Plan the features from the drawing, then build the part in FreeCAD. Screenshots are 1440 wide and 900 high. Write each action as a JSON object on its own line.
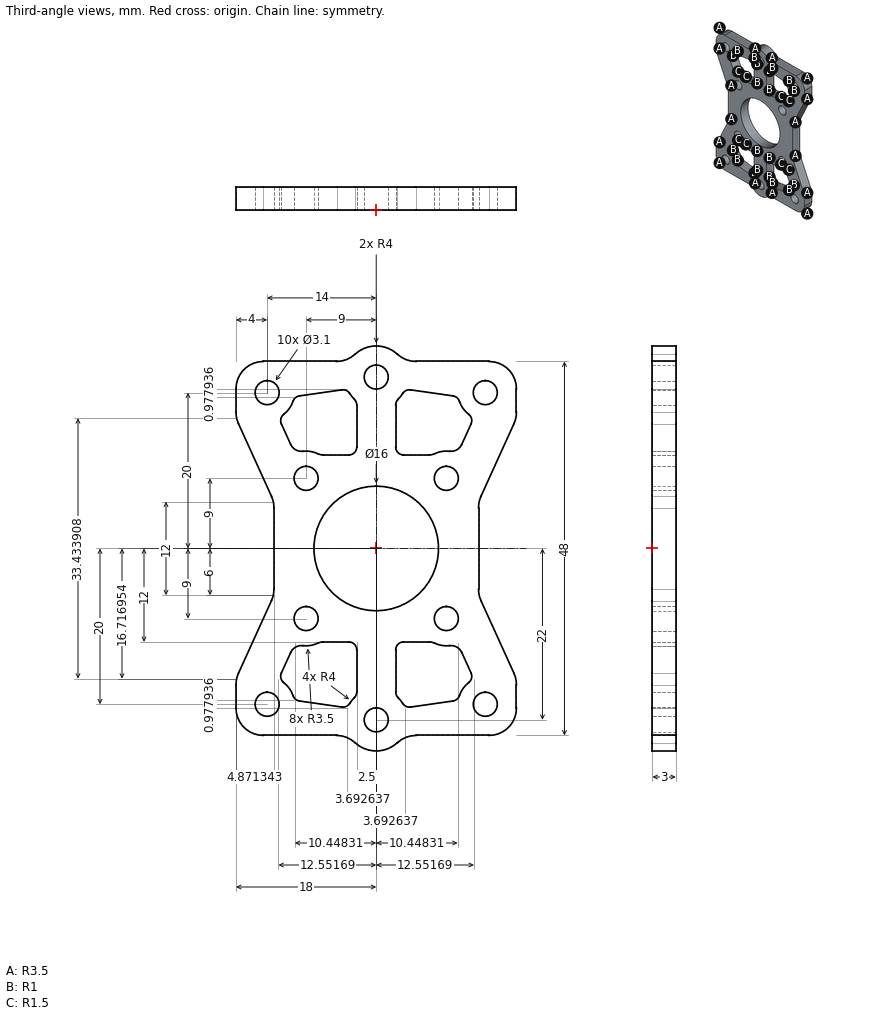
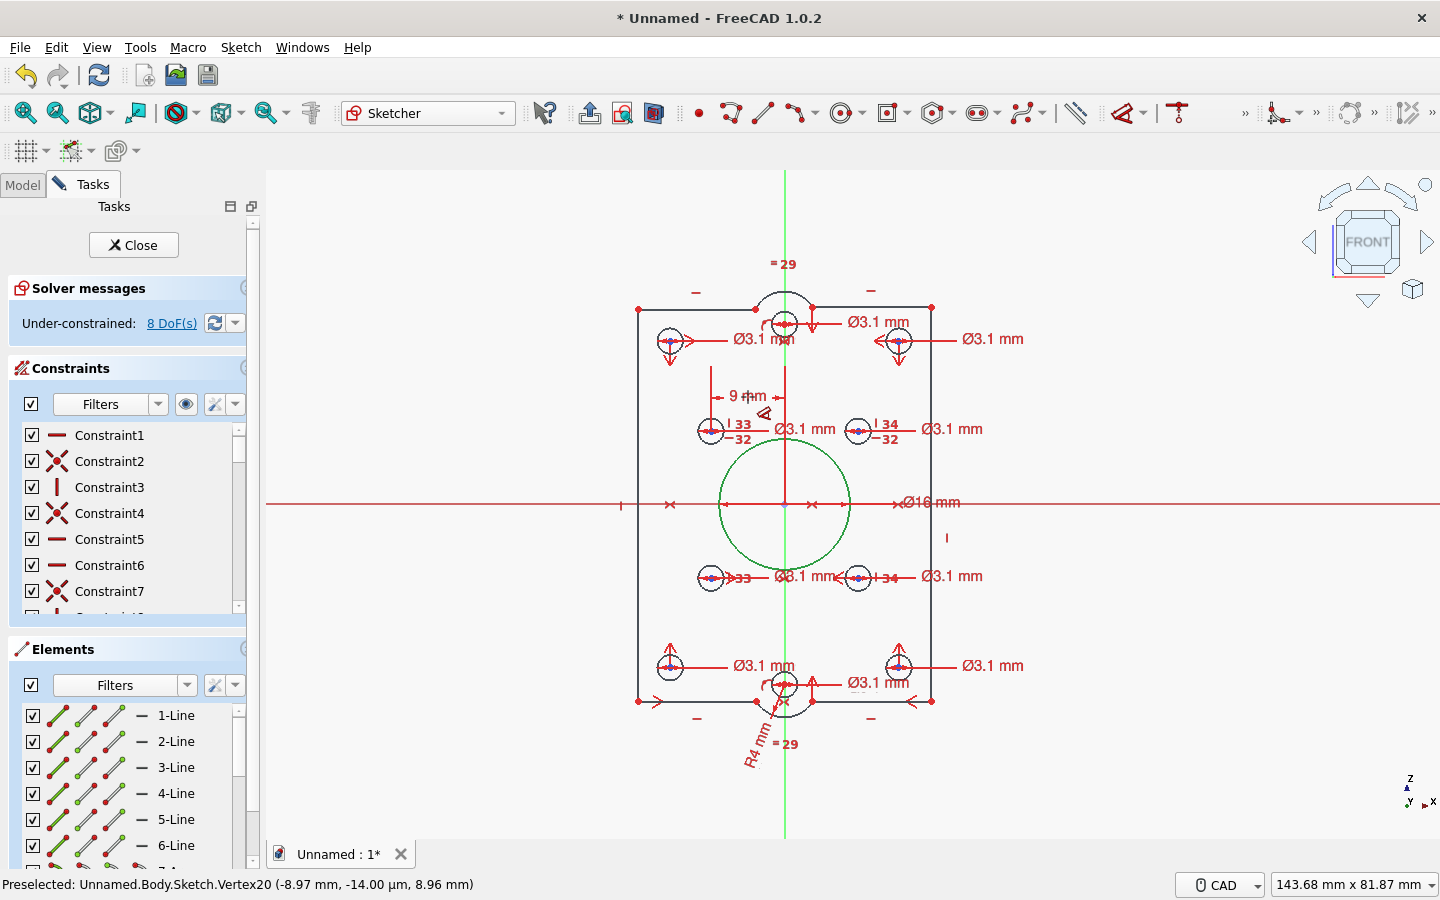
{"action": "left_click", "coordinate": [711, 431]}
{"action": "left_click", "coordinate": [677, 468]}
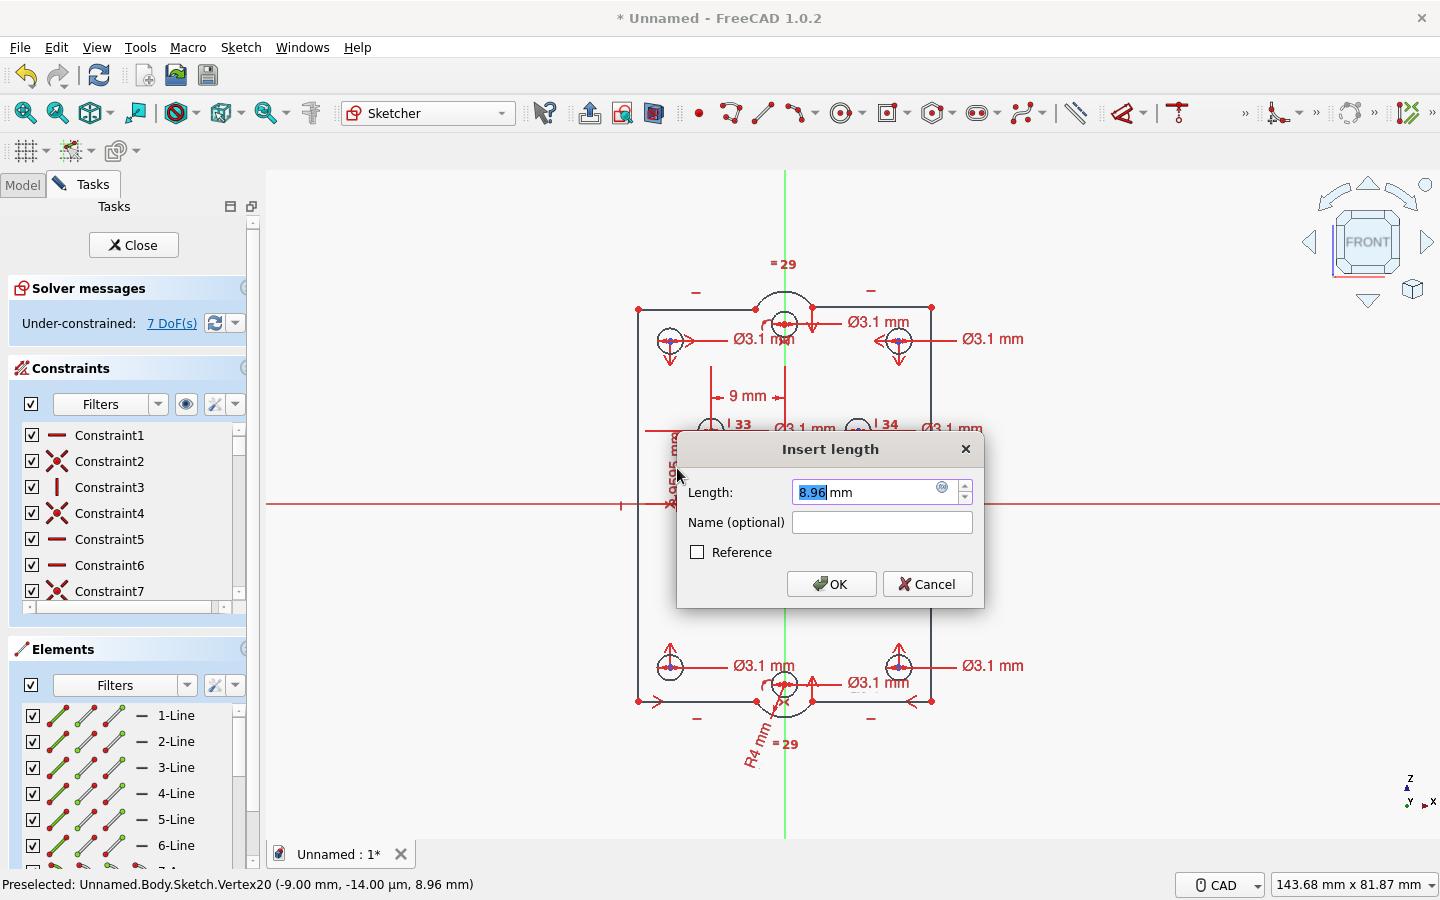
{"action": "type", "text": "9"}
{"action": "key", "text": "Return"}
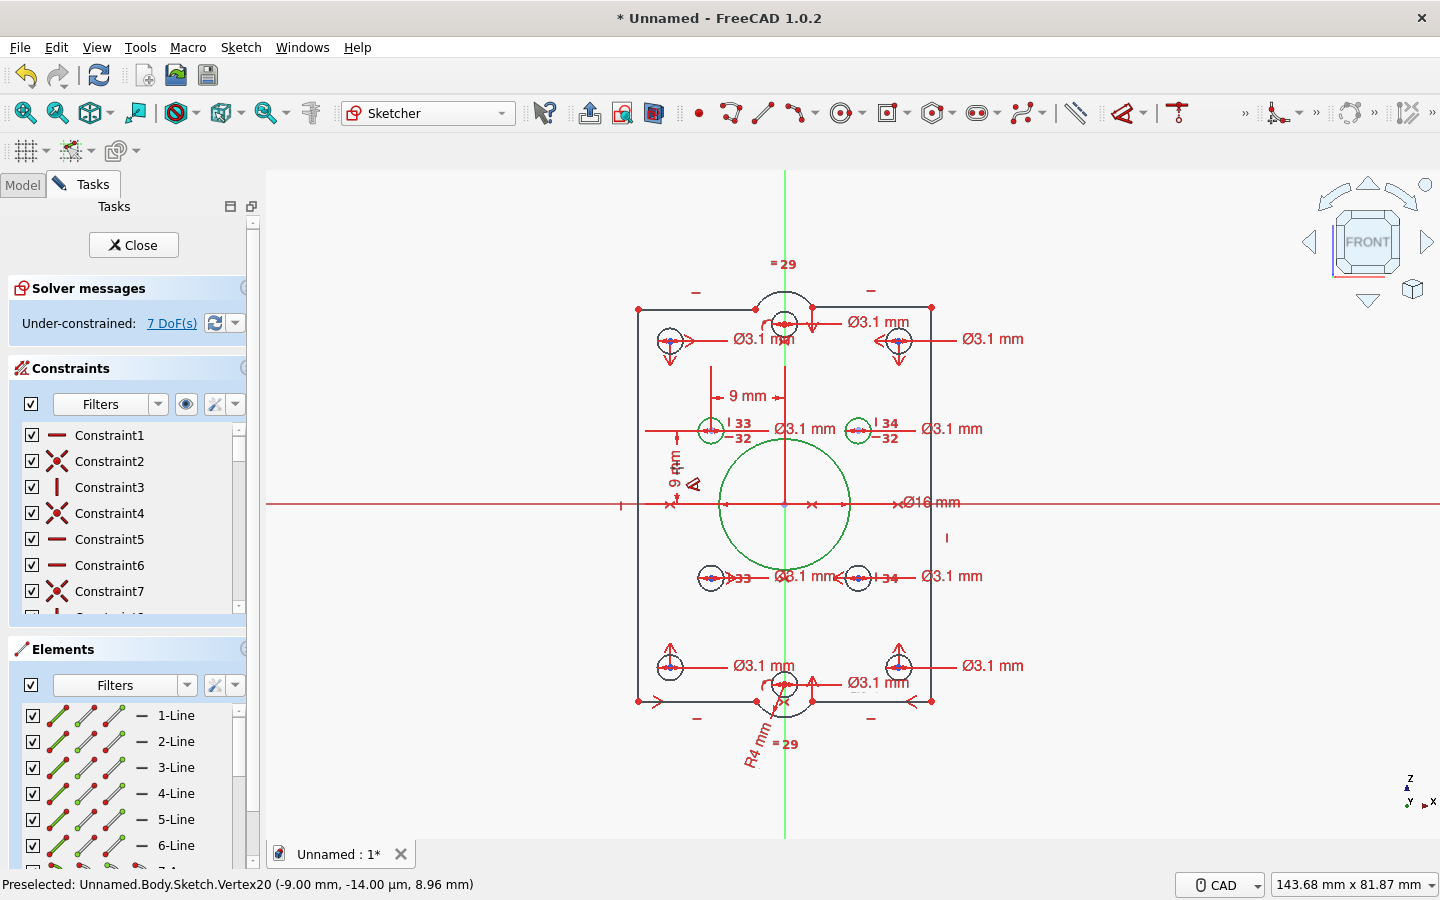
{"action": "left_click", "coordinate": [711, 578]}
{"action": "left_click", "coordinate": [677, 541]}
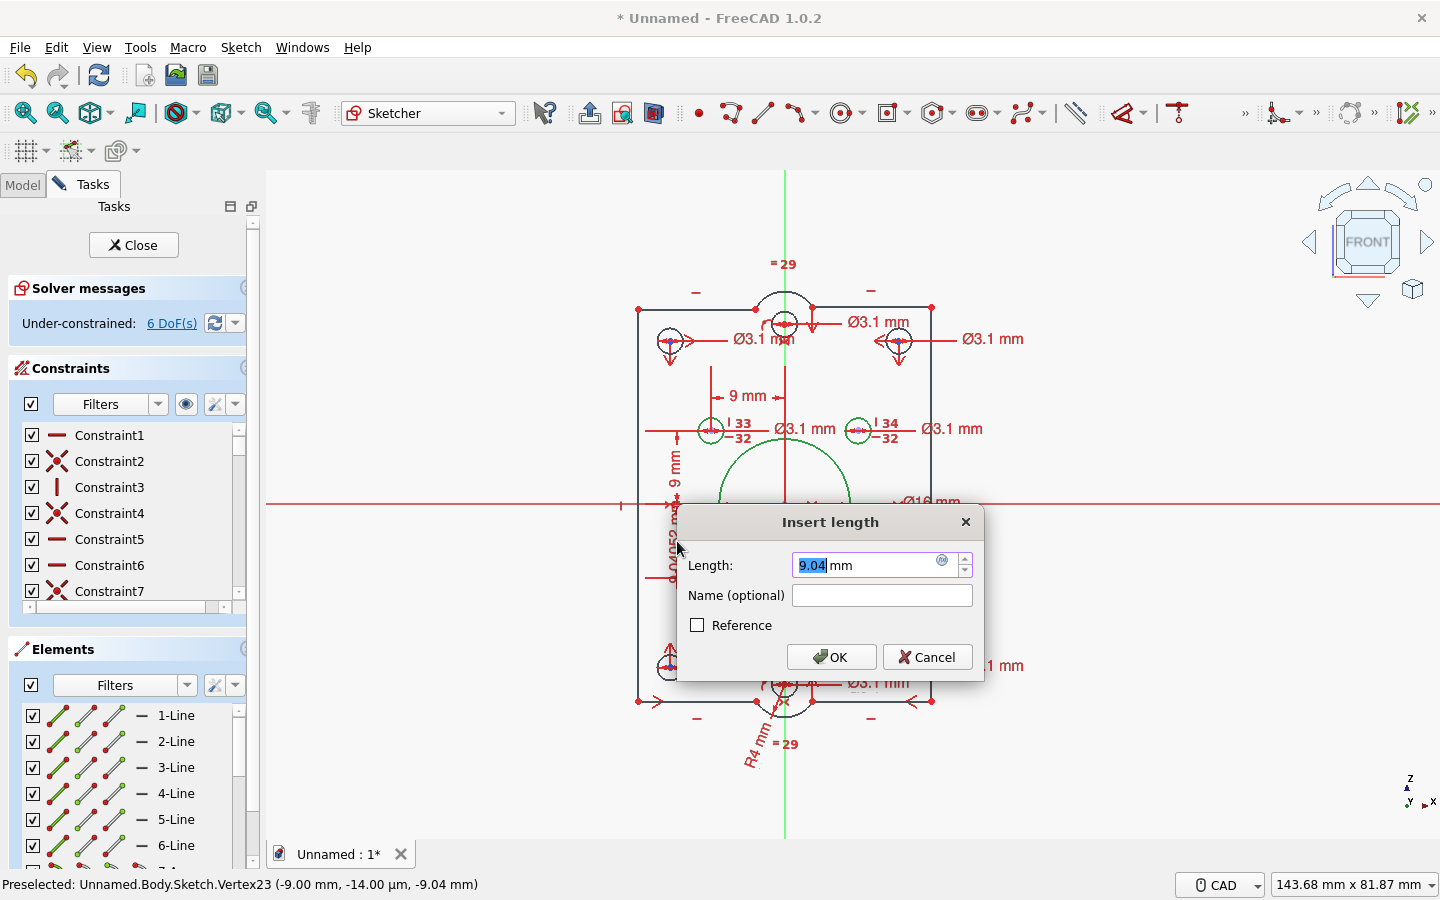
{"action": "type", "text": "9"}
{"action": "key", "text": "Return"}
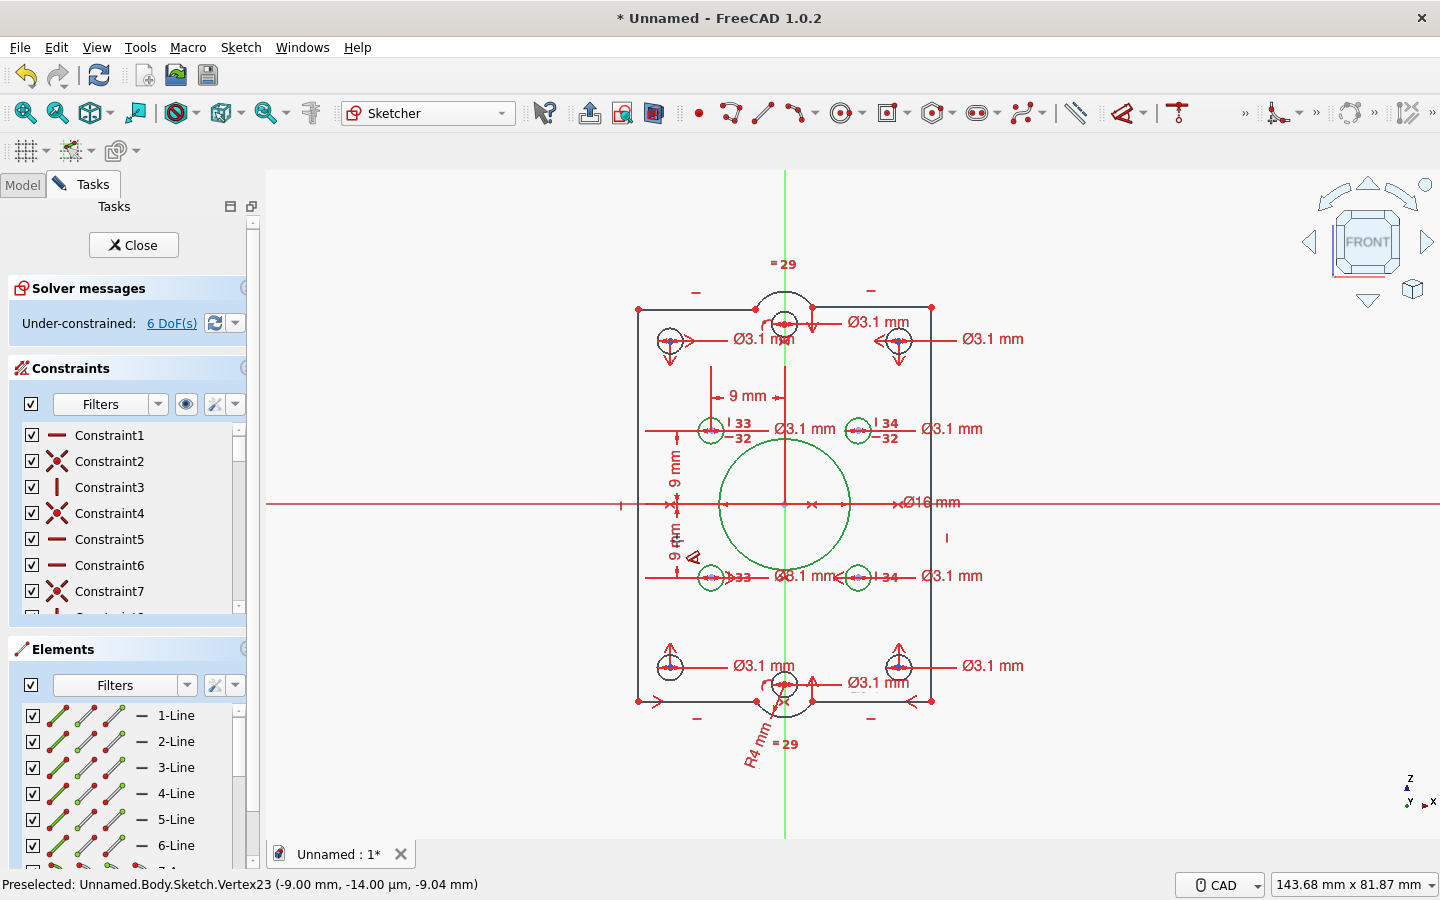
{"action": "left_click", "coordinate": [931, 426]}
{"action": "left_click", "coordinate": [965, 414]}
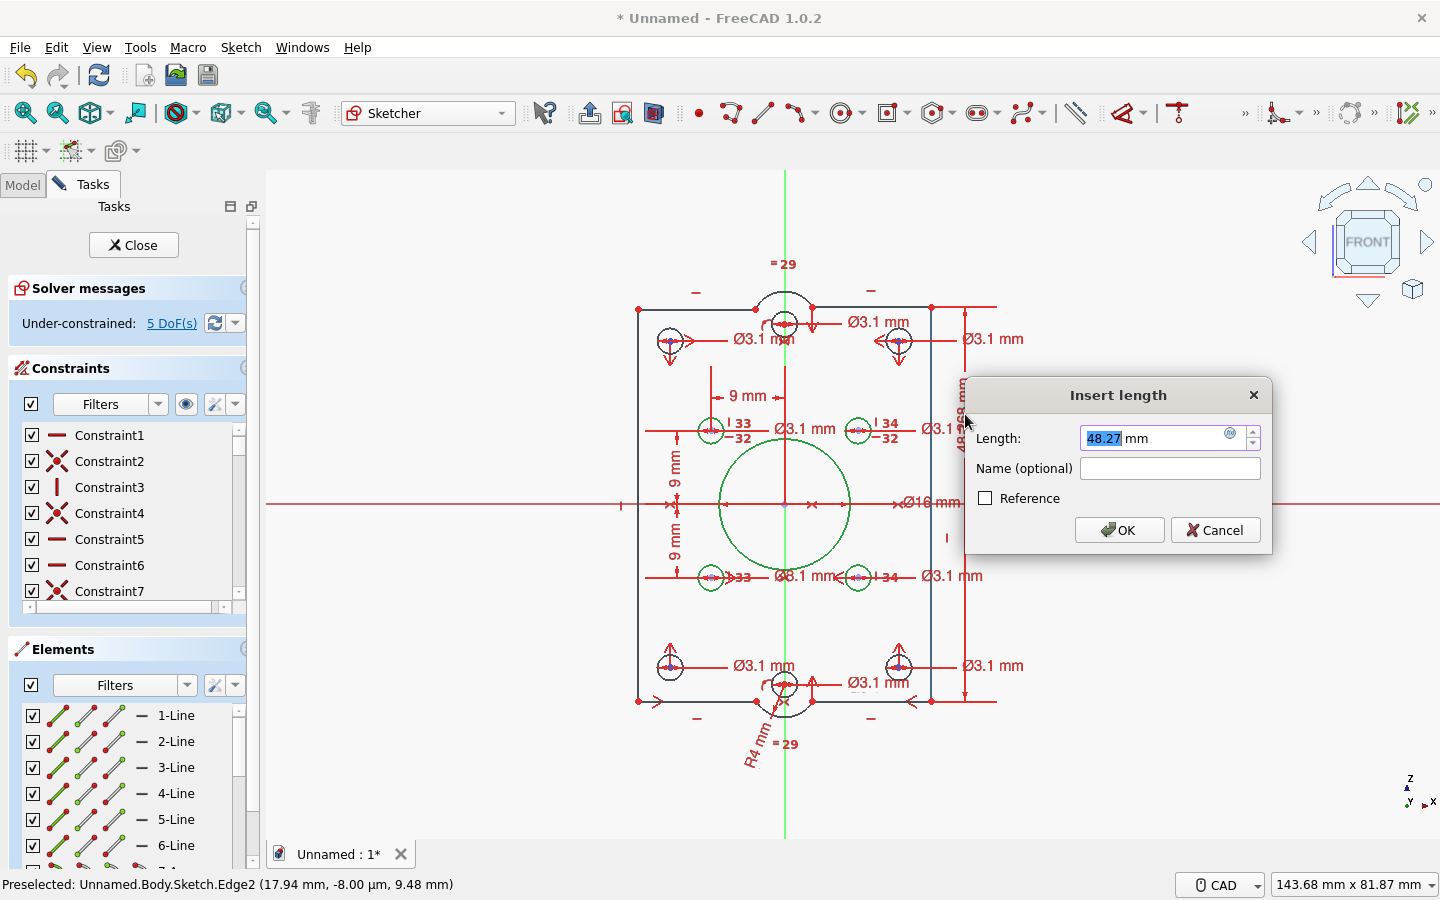
{"action": "type", "text": "48"}
{"action": "key", "text": "Return"}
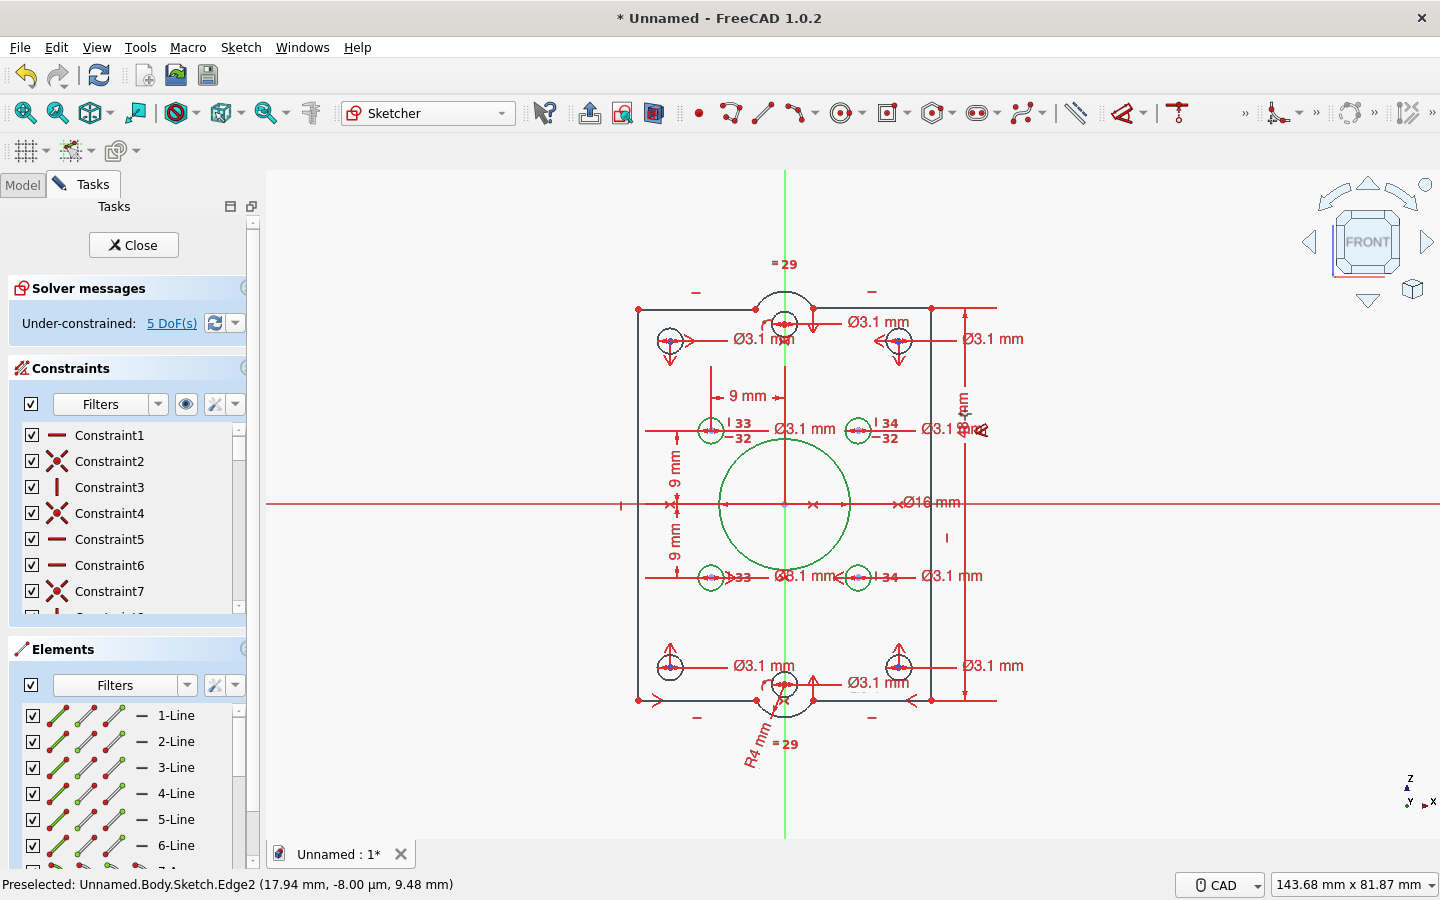
{"action": "left_click", "coordinate": [638, 583]}
{"action": "left_click", "coordinate": [604, 415]}